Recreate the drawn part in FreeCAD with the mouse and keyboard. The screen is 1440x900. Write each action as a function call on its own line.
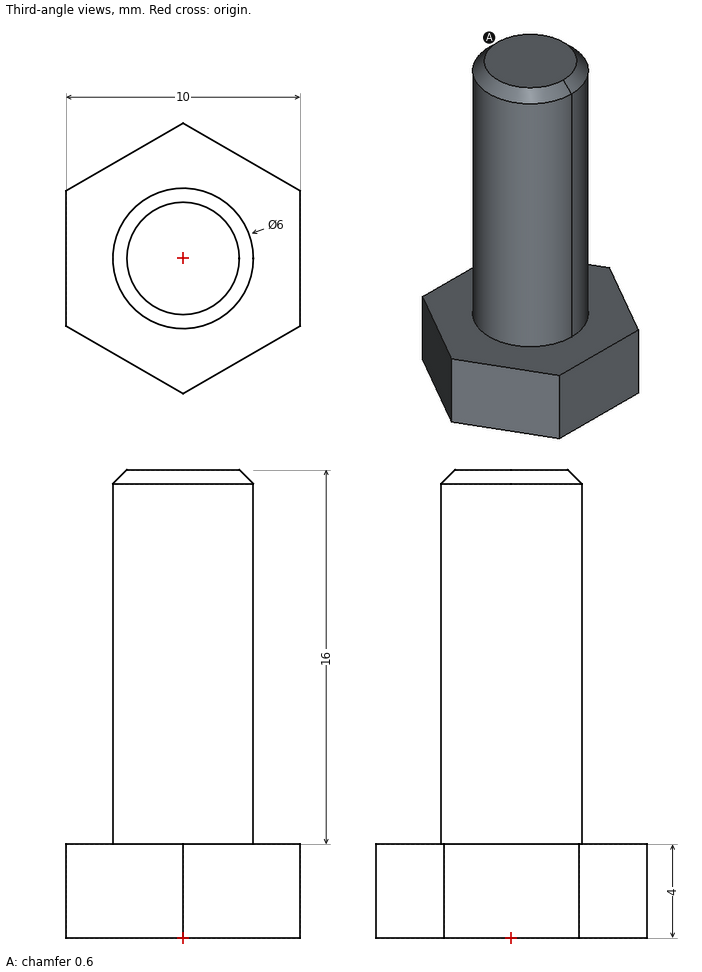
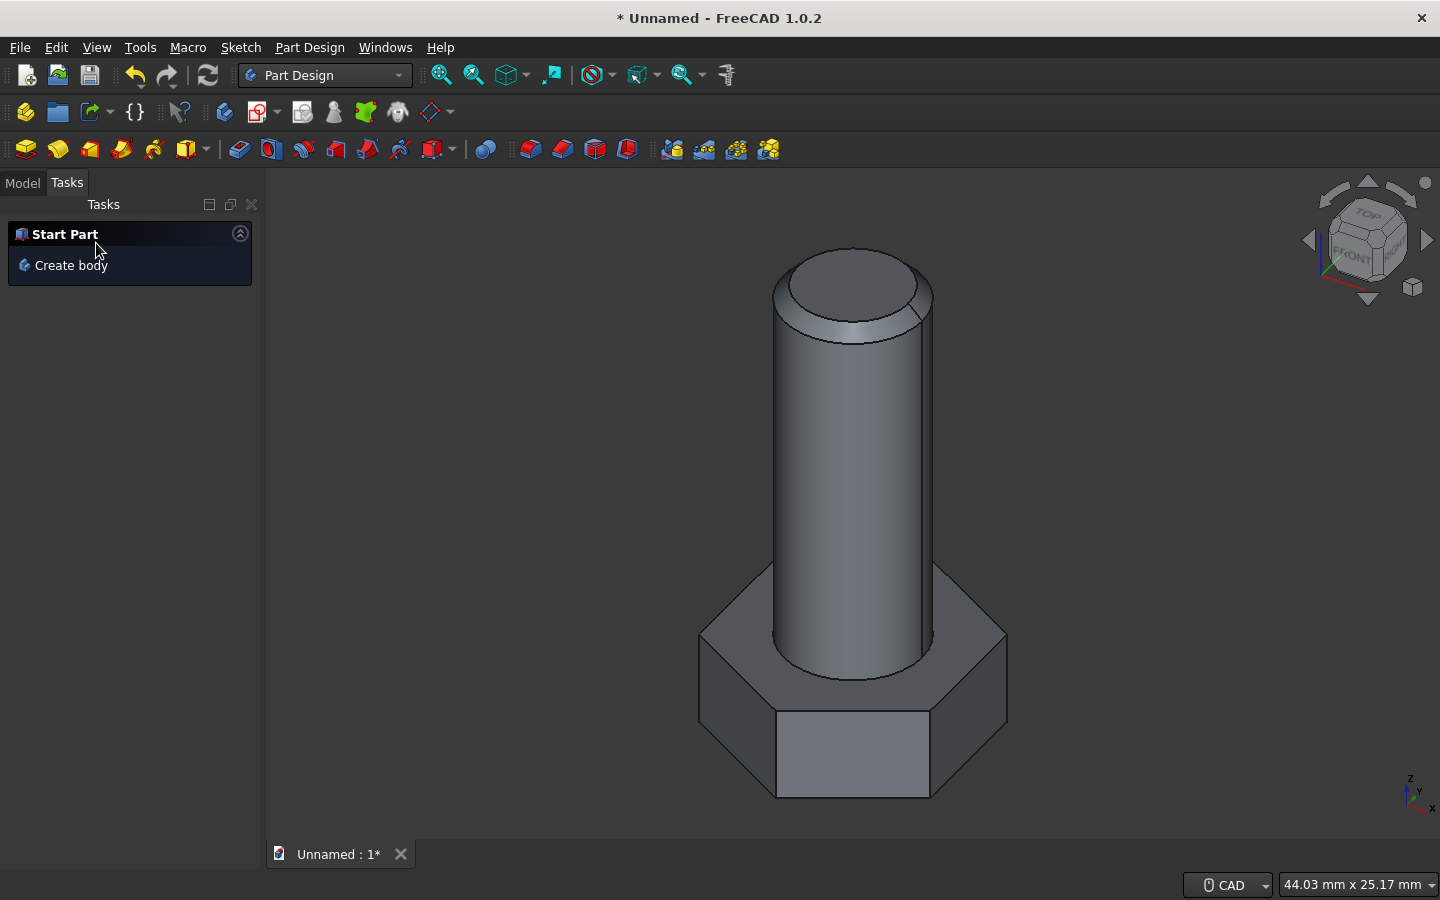
key(0)